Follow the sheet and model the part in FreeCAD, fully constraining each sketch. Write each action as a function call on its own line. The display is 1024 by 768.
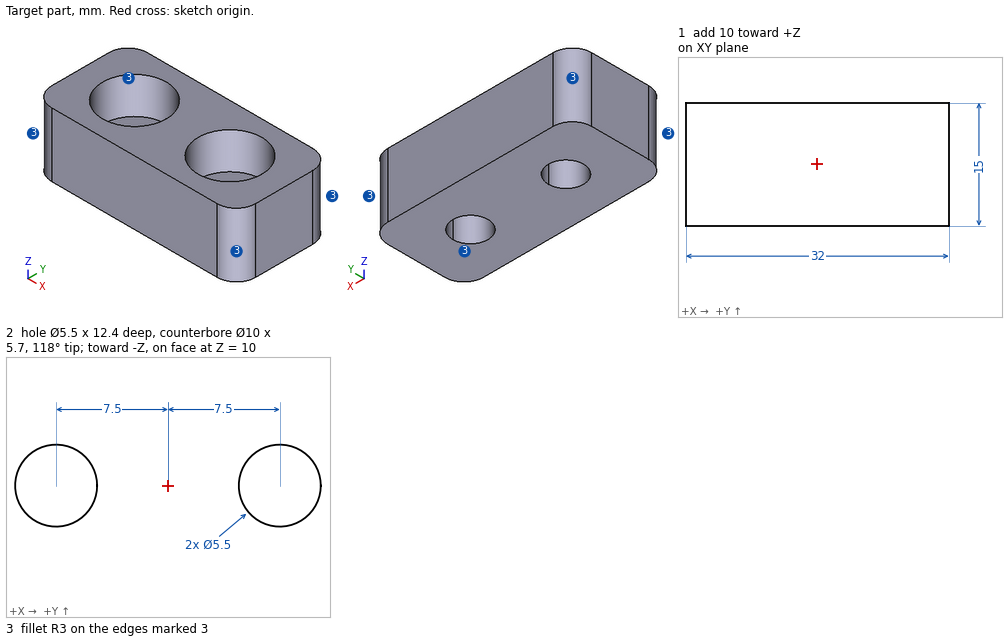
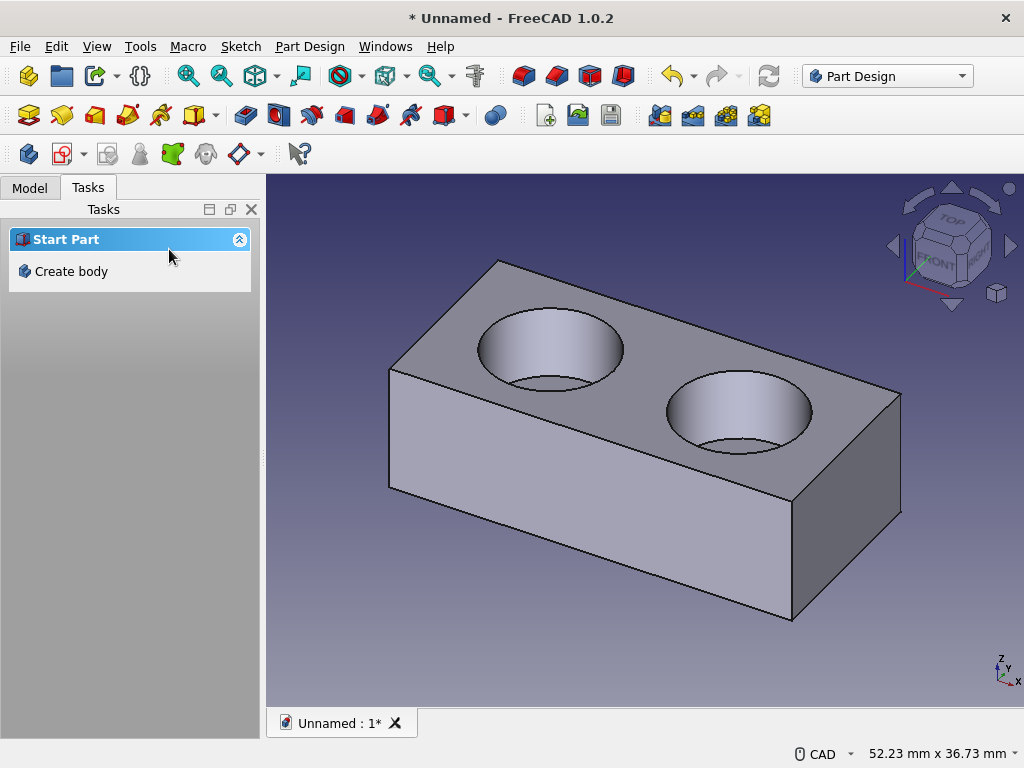
click(792, 560)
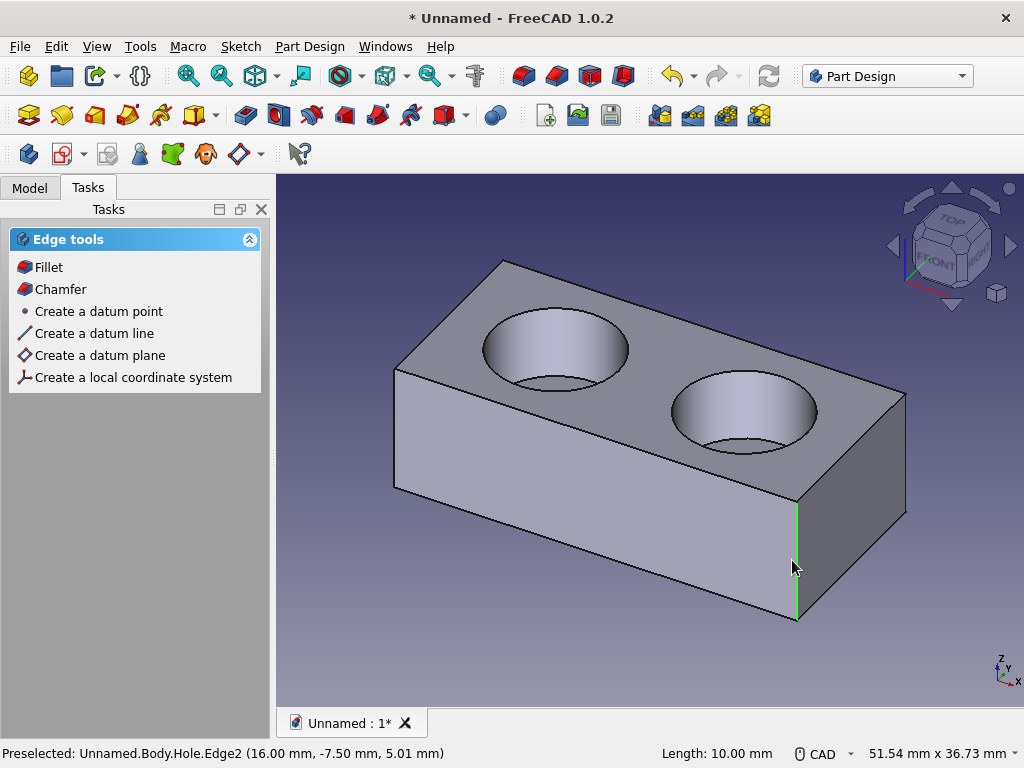
key(0)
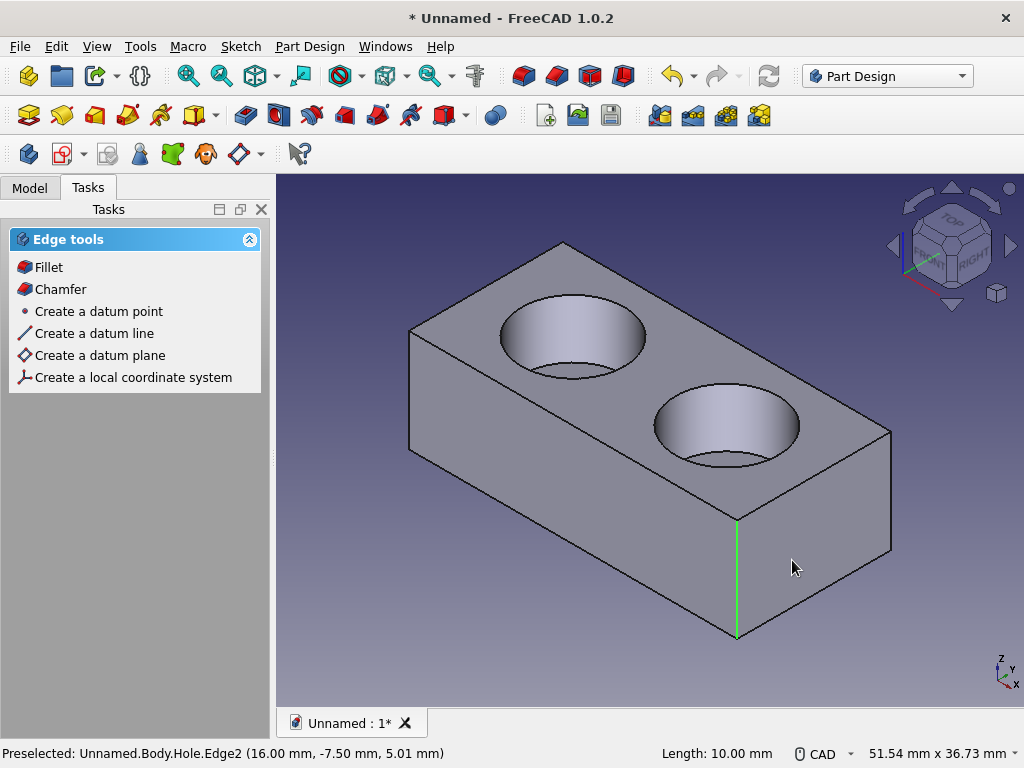
key(2)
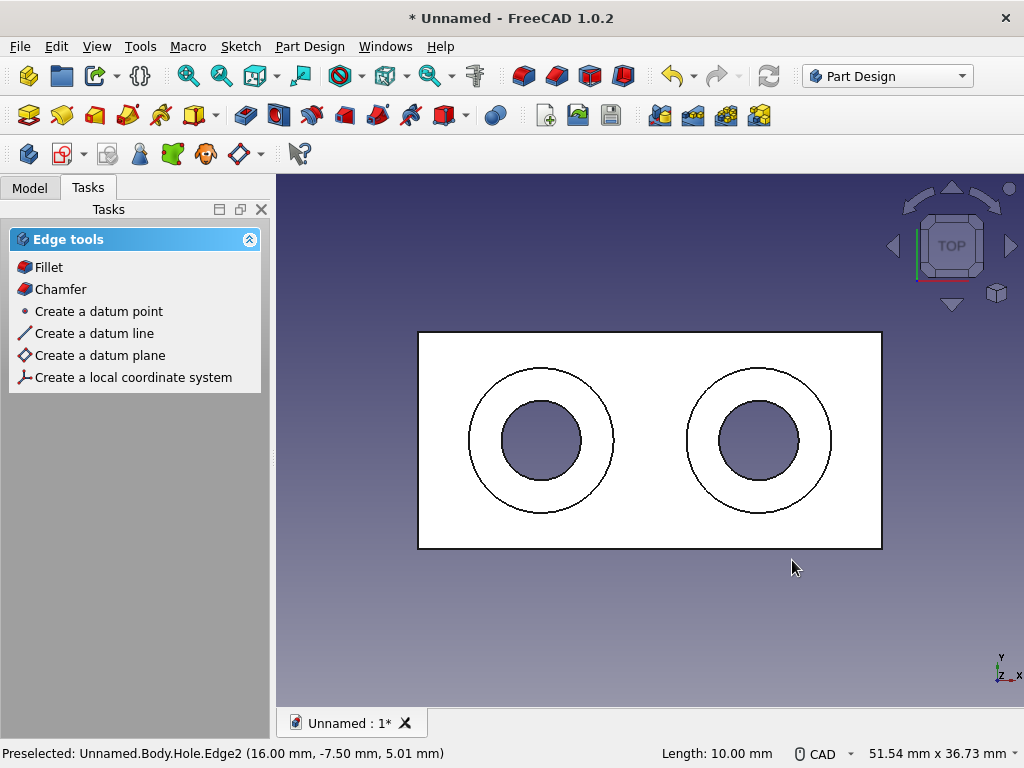
key(1)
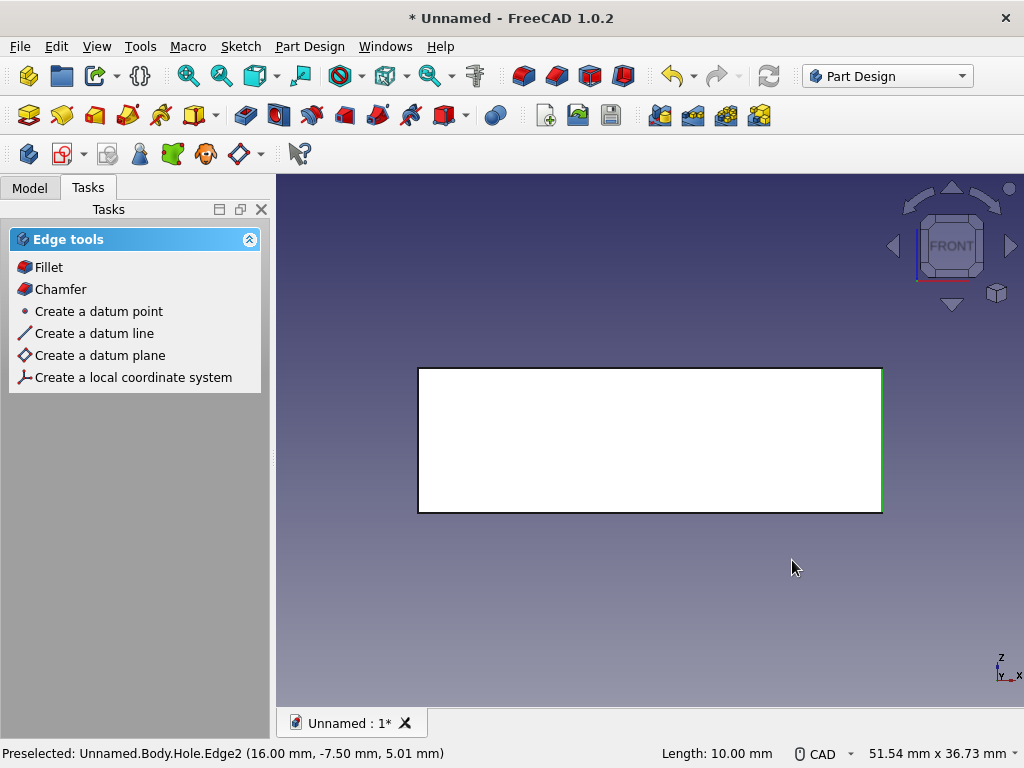
click(418, 440, ctrl)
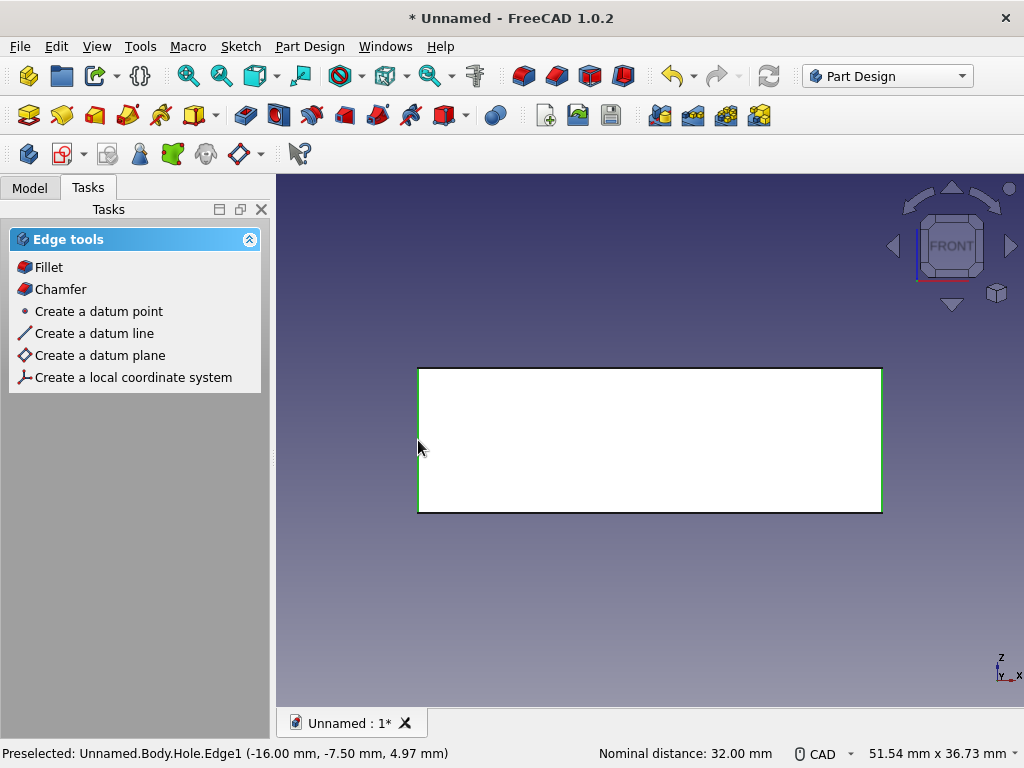
key(3)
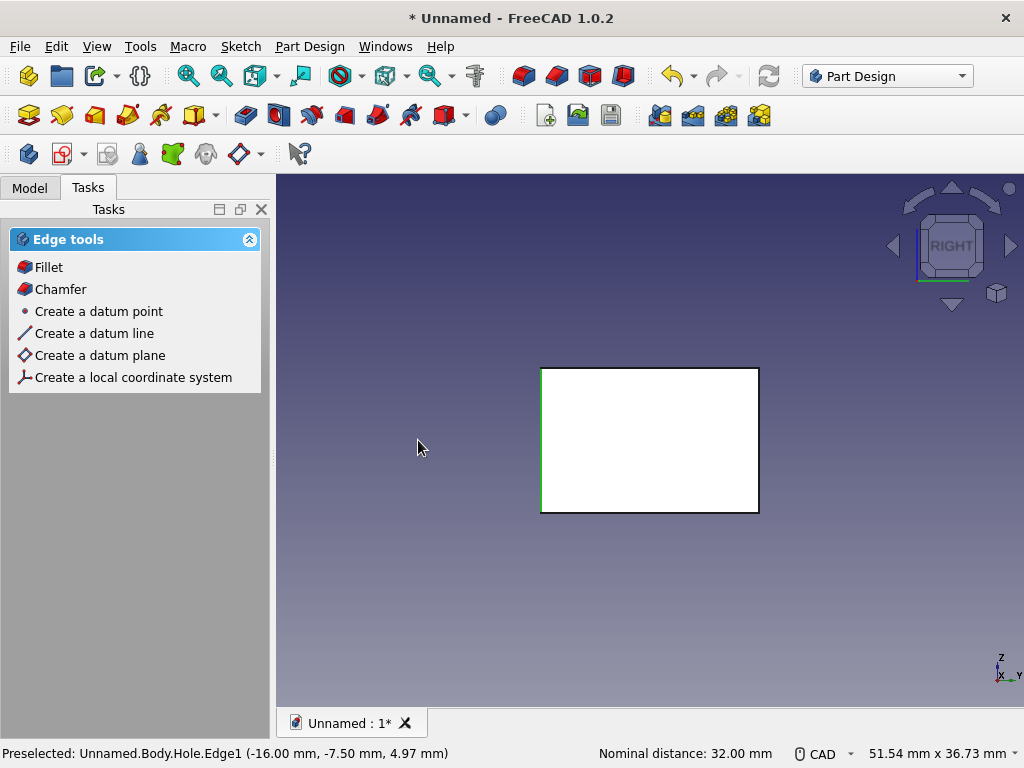
key(v)
key(f)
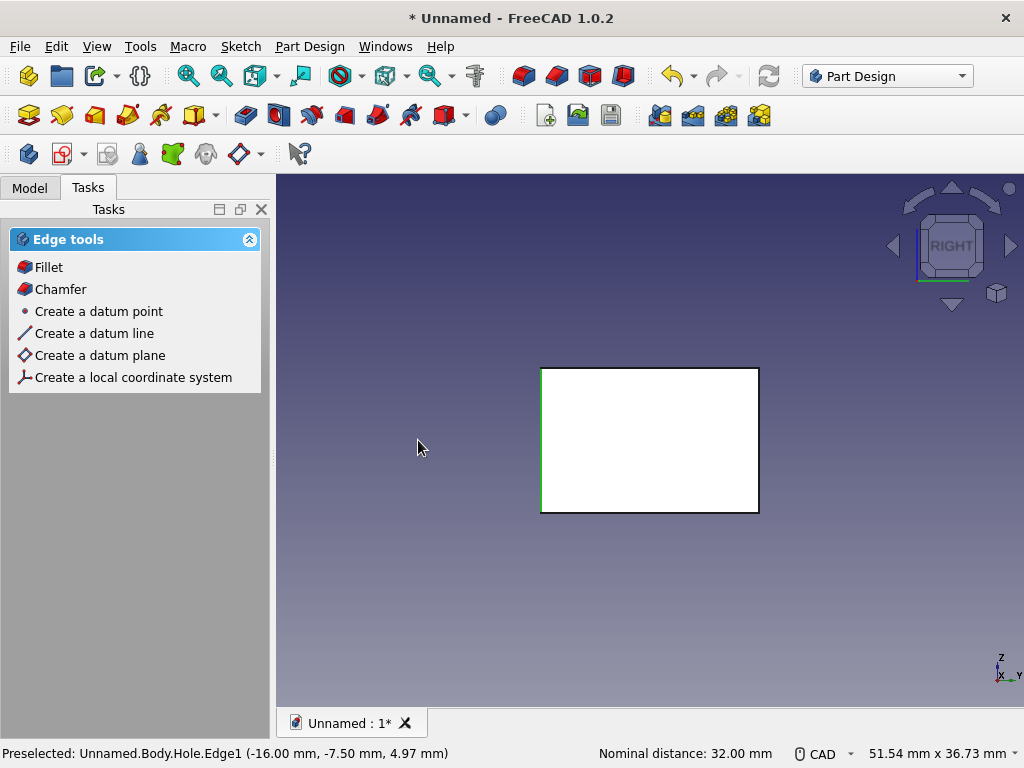
click(759, 439, ctrl)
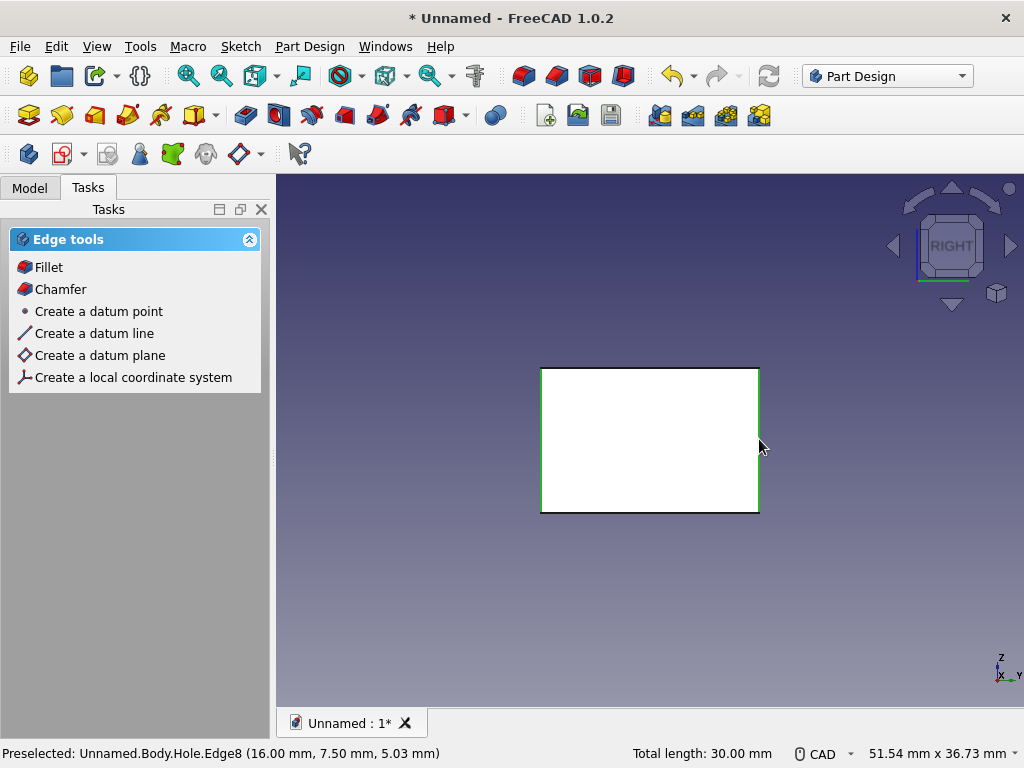
key(5)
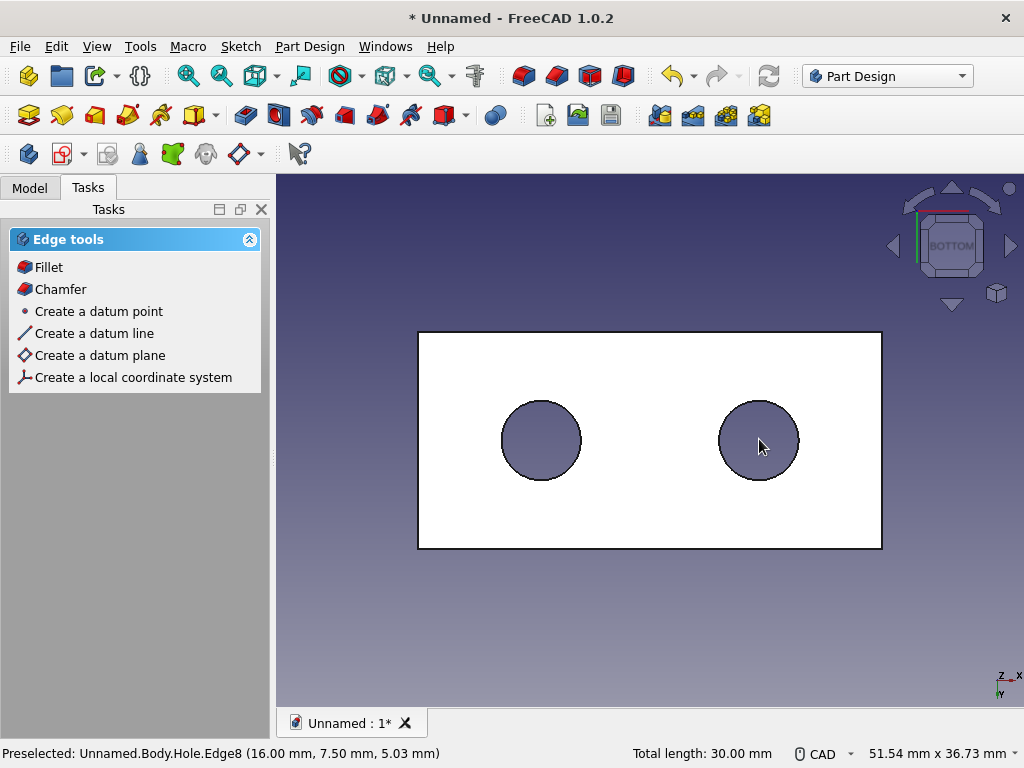
key(4)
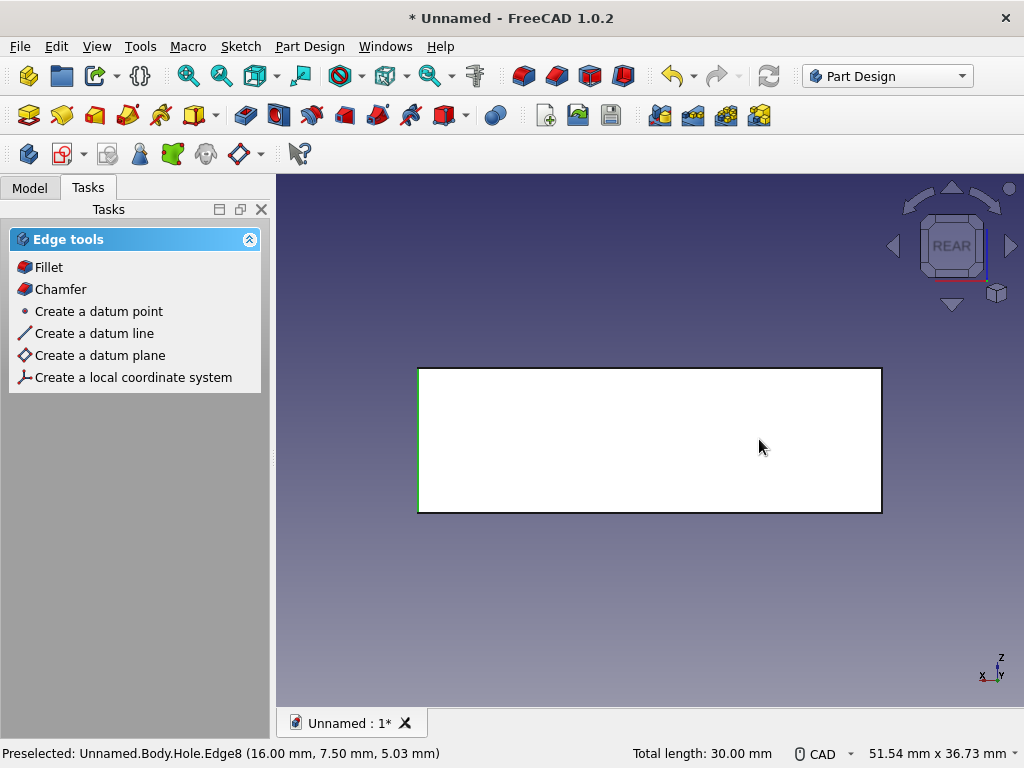
click(882, 440, ctrl)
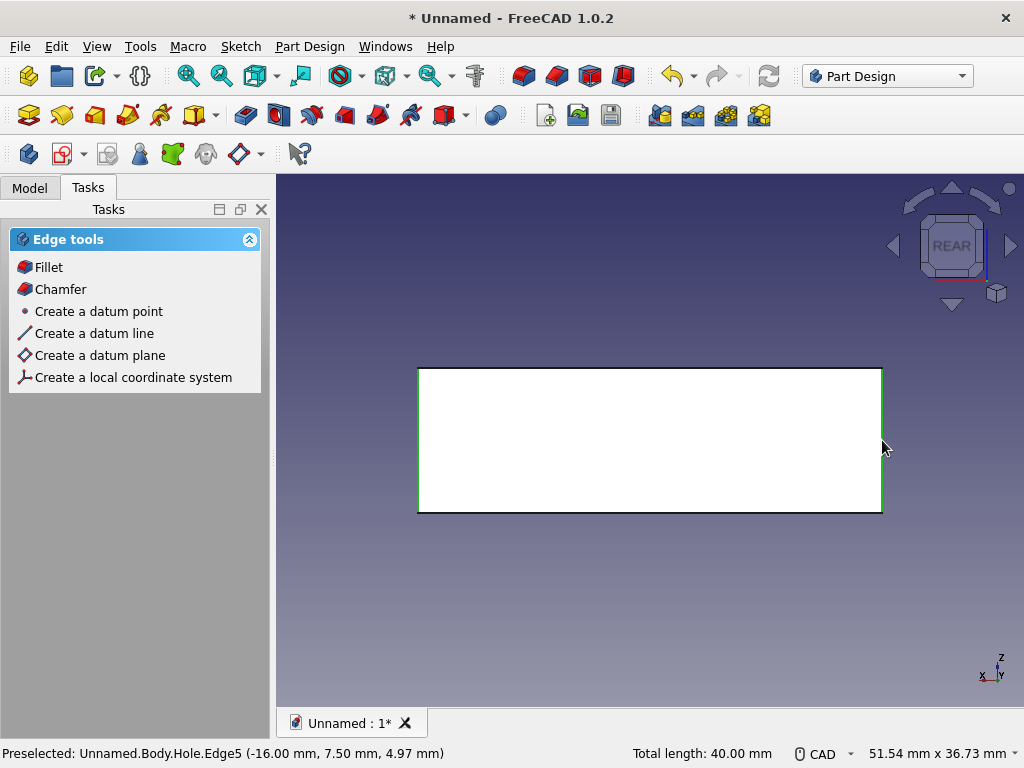
click(524, 76)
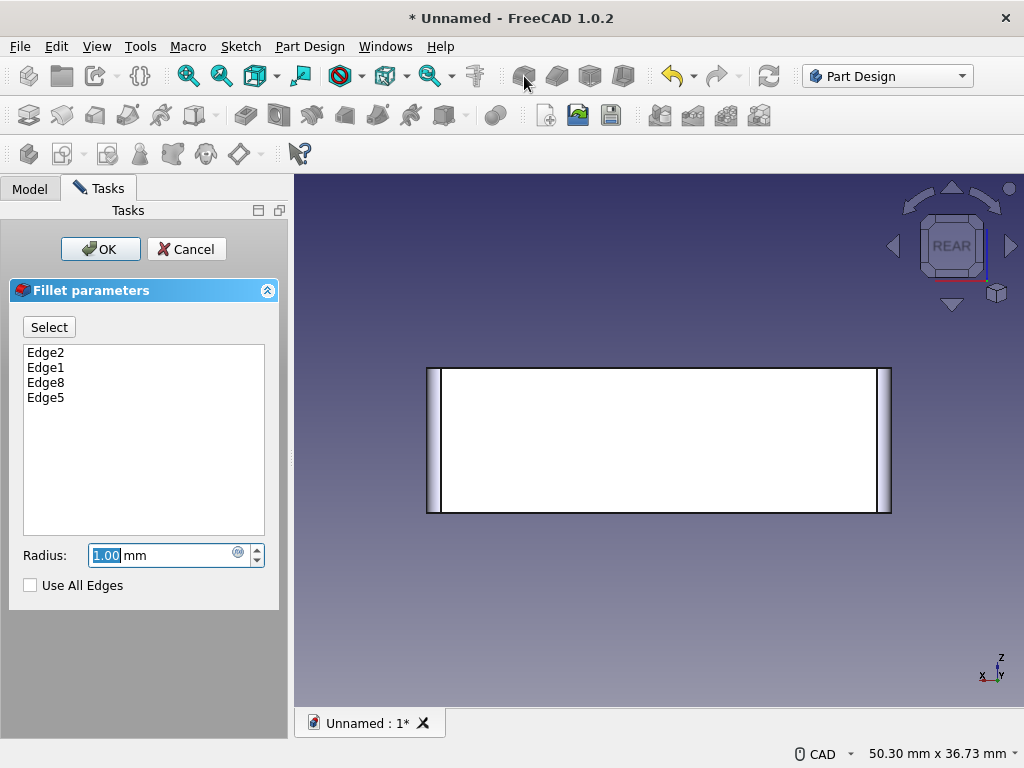
text(3)
key(Tab)